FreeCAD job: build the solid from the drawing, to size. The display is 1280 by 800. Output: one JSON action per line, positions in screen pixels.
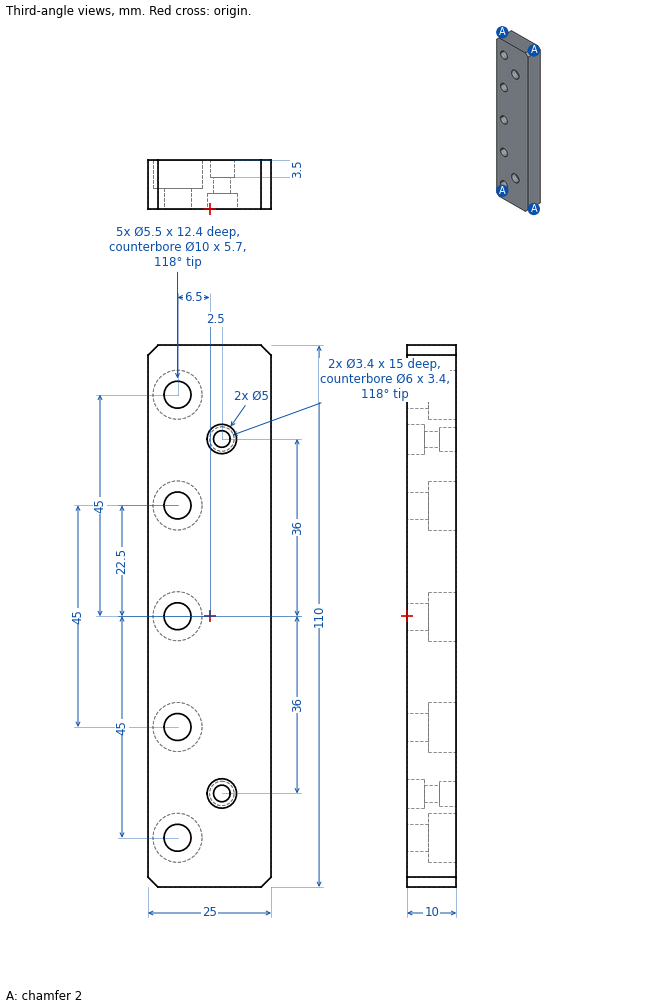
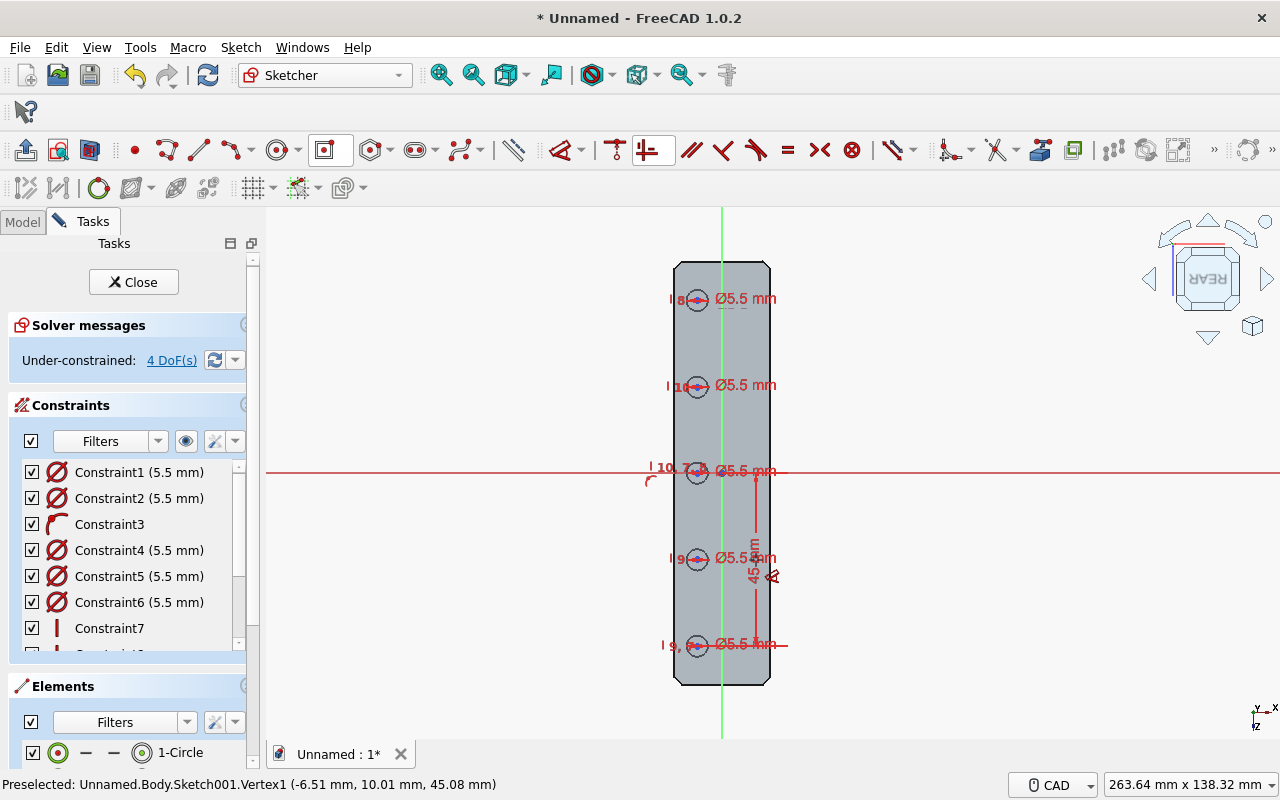
{"action": "left_click", "coordinate": [697, 301]}
{"action": "left_click", "coordinate": [756, 387]}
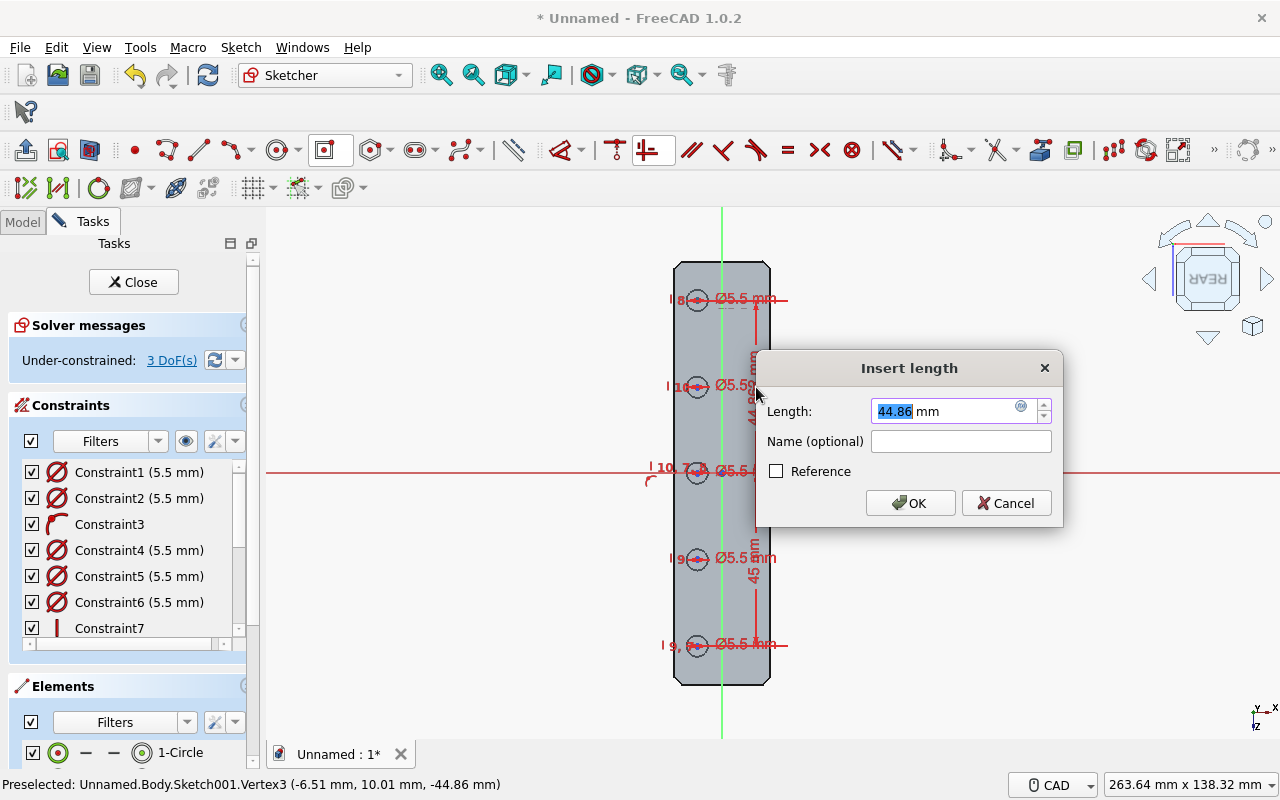
{"action": "type", "text": "45"}
{"action": "key", "text": "Return"}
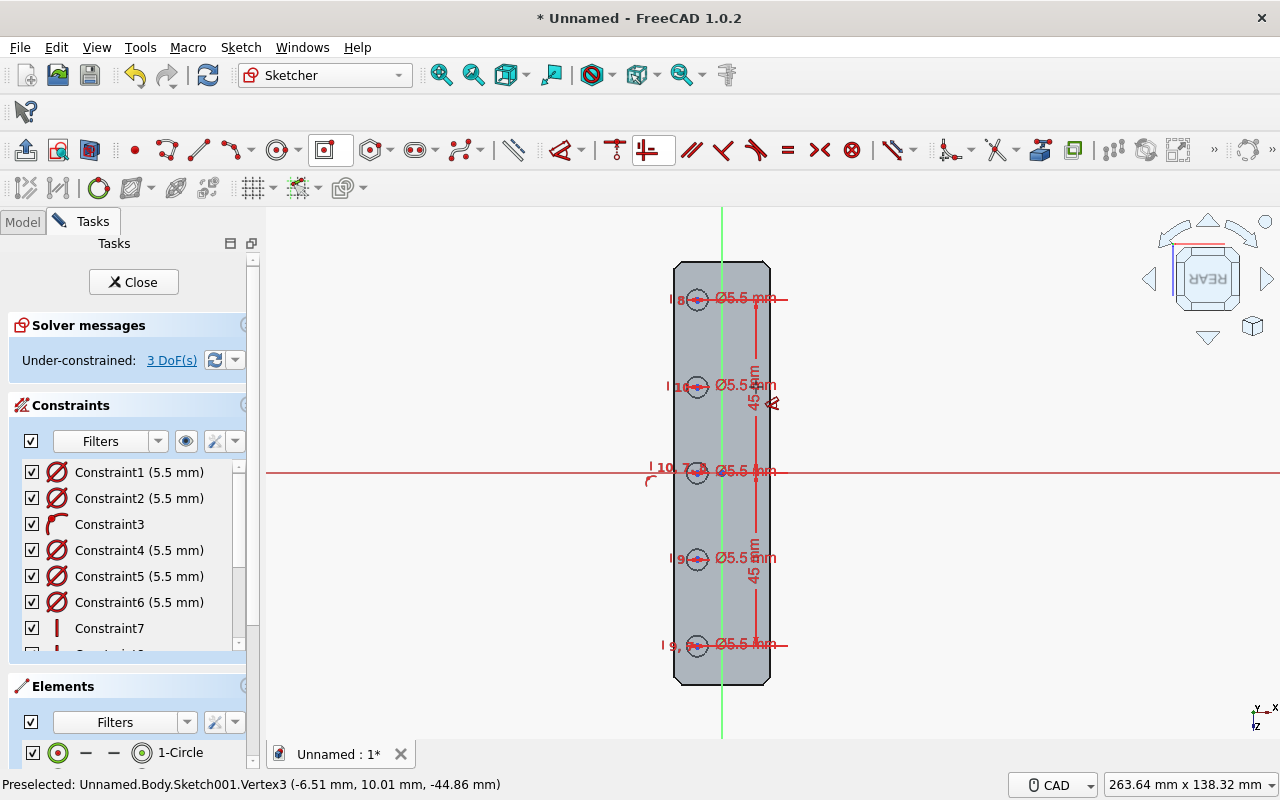
{"action": "scroll", "coordinate": [697, 646], "scroll_direction": "up", "scroll_amount": 3}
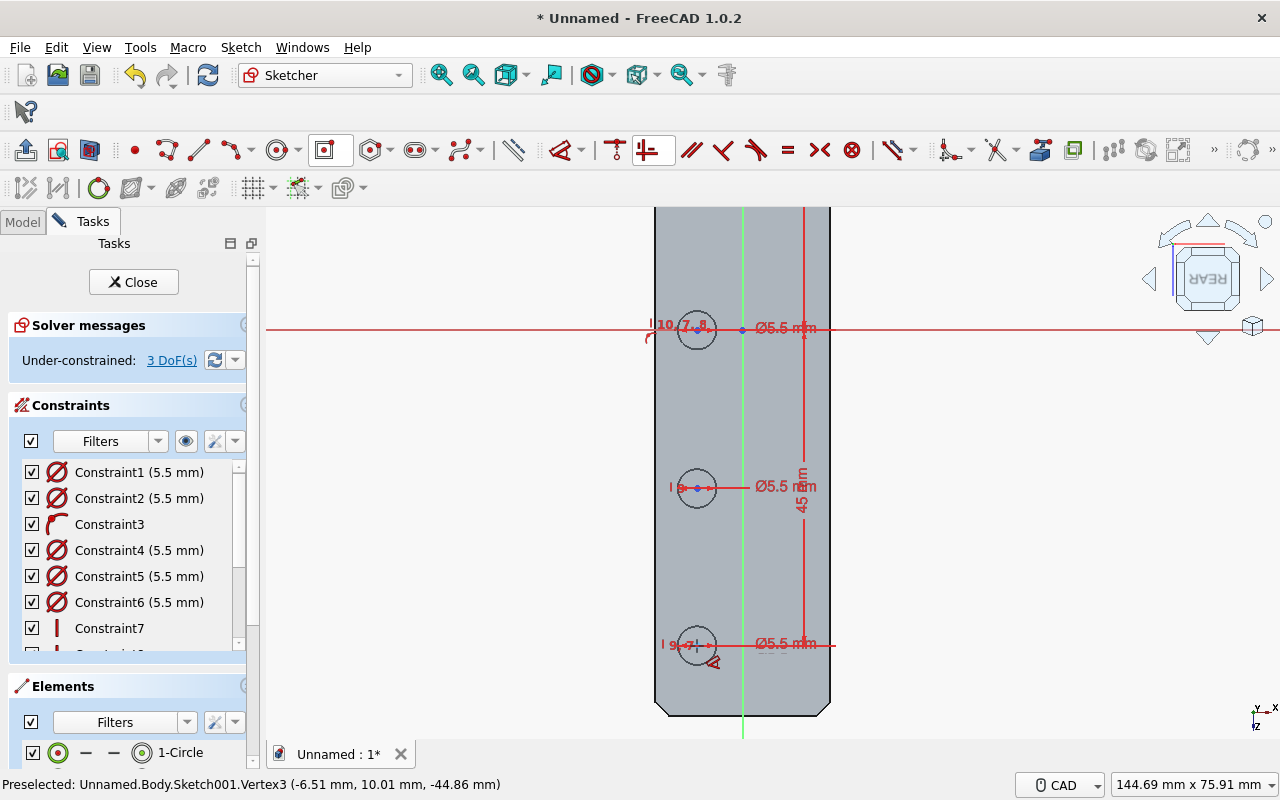
{"action": "left_click", "coordinate": [697, 646]}
{"action": "left_click", "coordinate": [720, 680]}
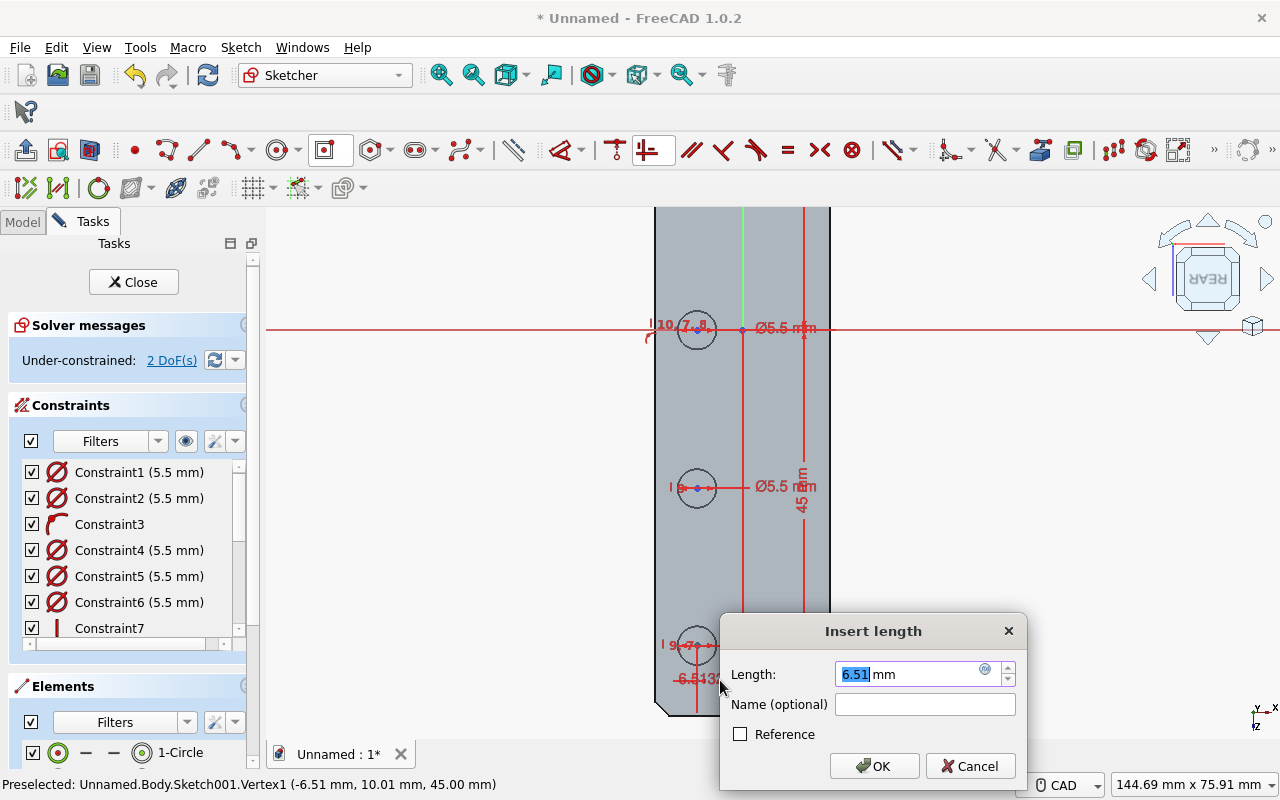
{"action": "type", "text": "6.5"}
{"action": "key", "text": "Return"}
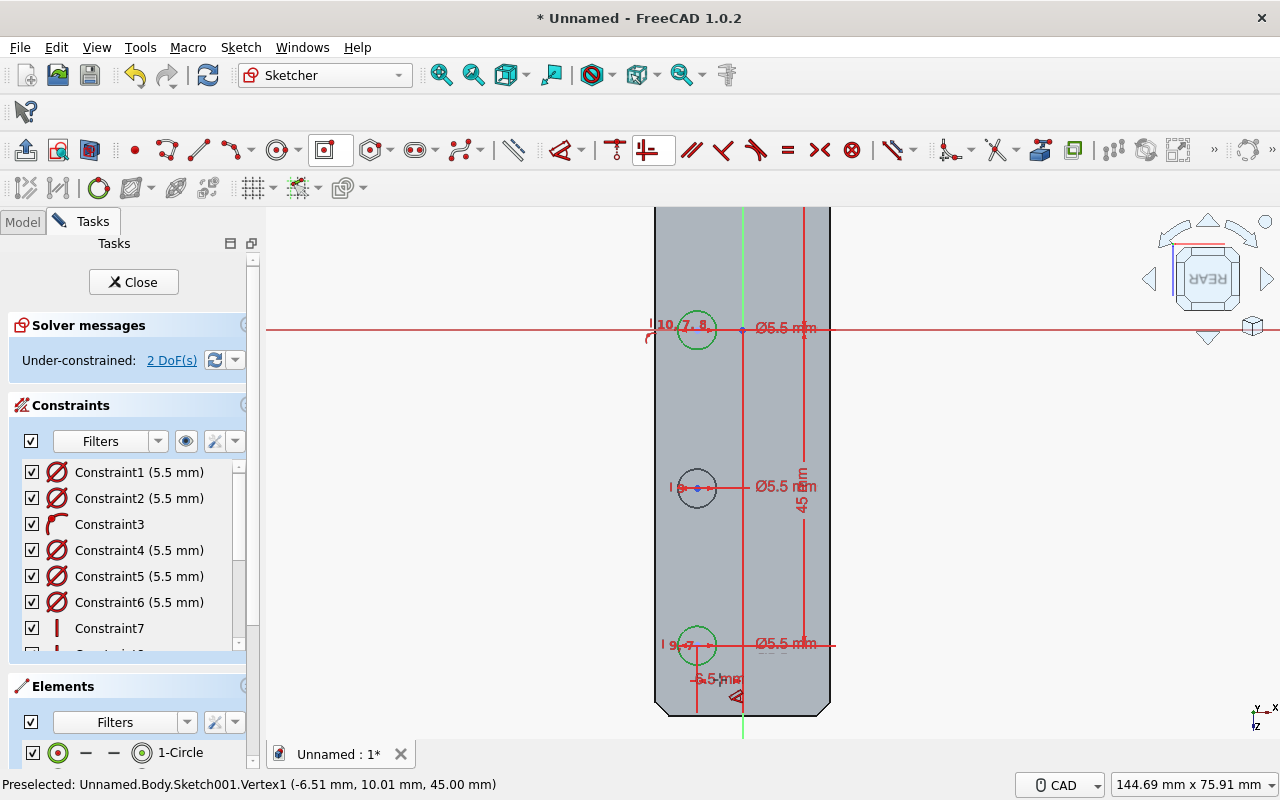
{"action": "left_click", "coordinate": [697, 488]}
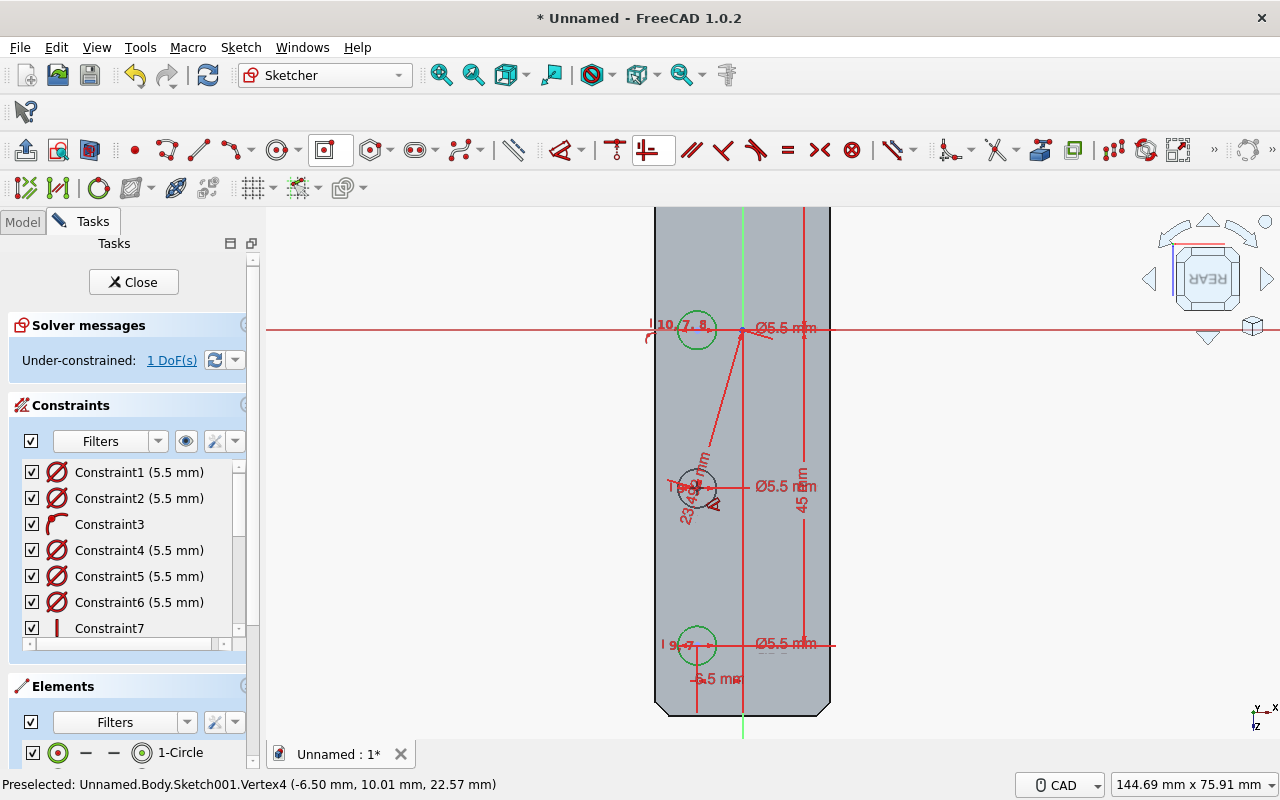
{"action": "scroll", "coordinate": [697, 647], "scroll_direction": "down", "scroll_amount": 3}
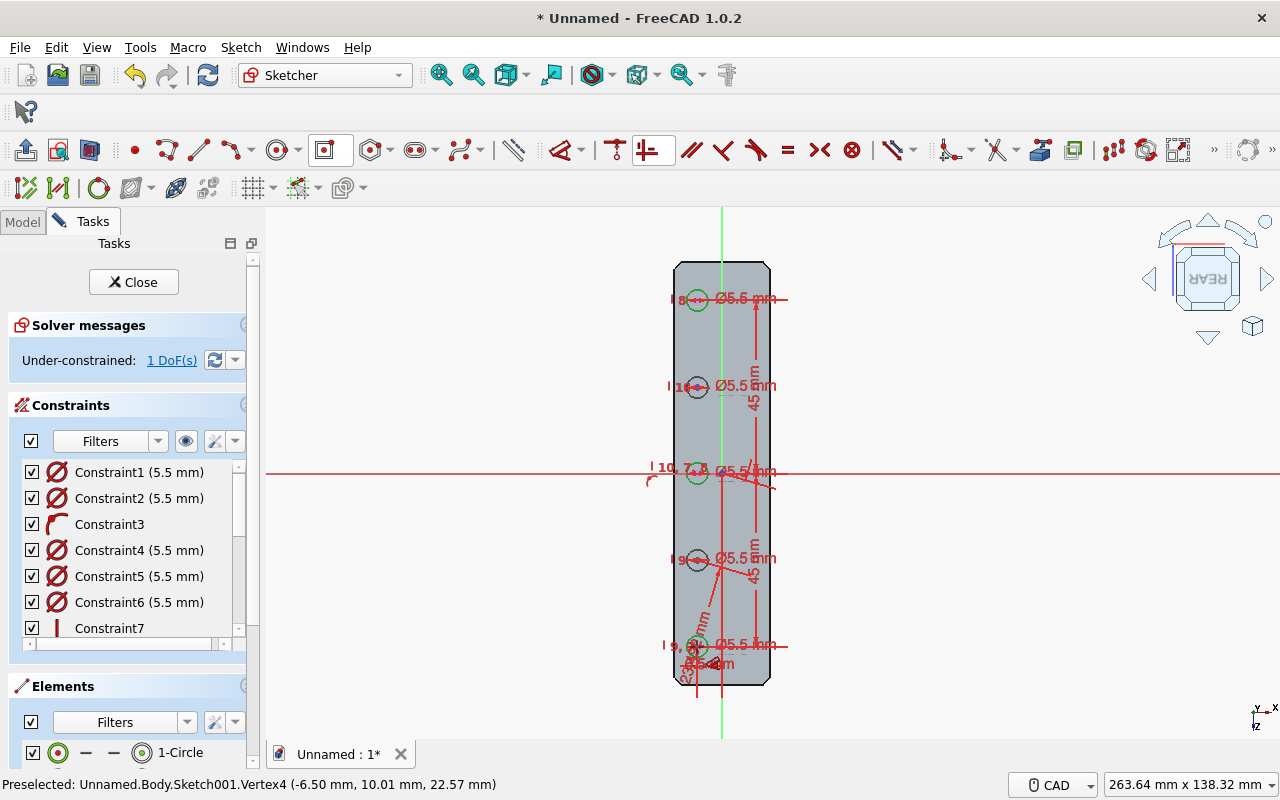
{"action": "left_click", "coordinate": [697, 388]}
{"action": "left_click", "coordinate": [663, 434]}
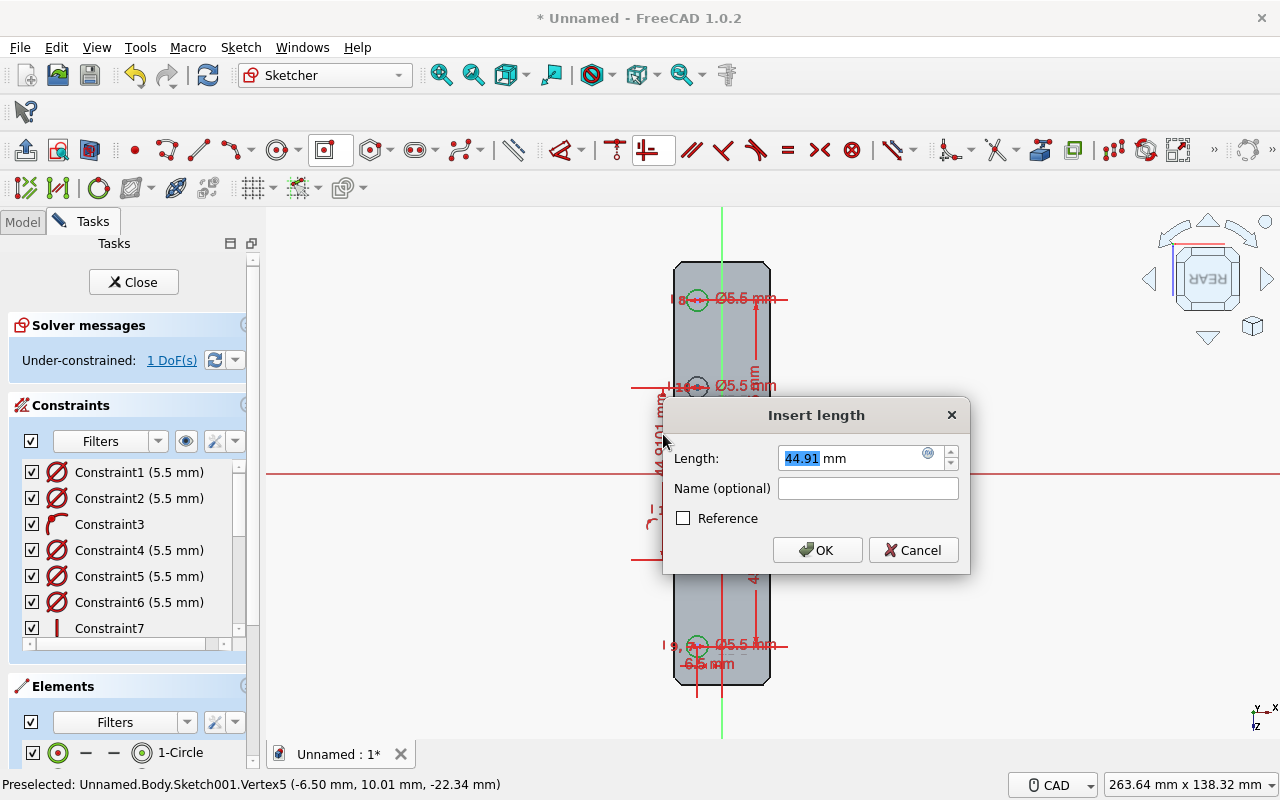
{"action": "type", "text": "45"}
{"action": "key", "text": "Return"}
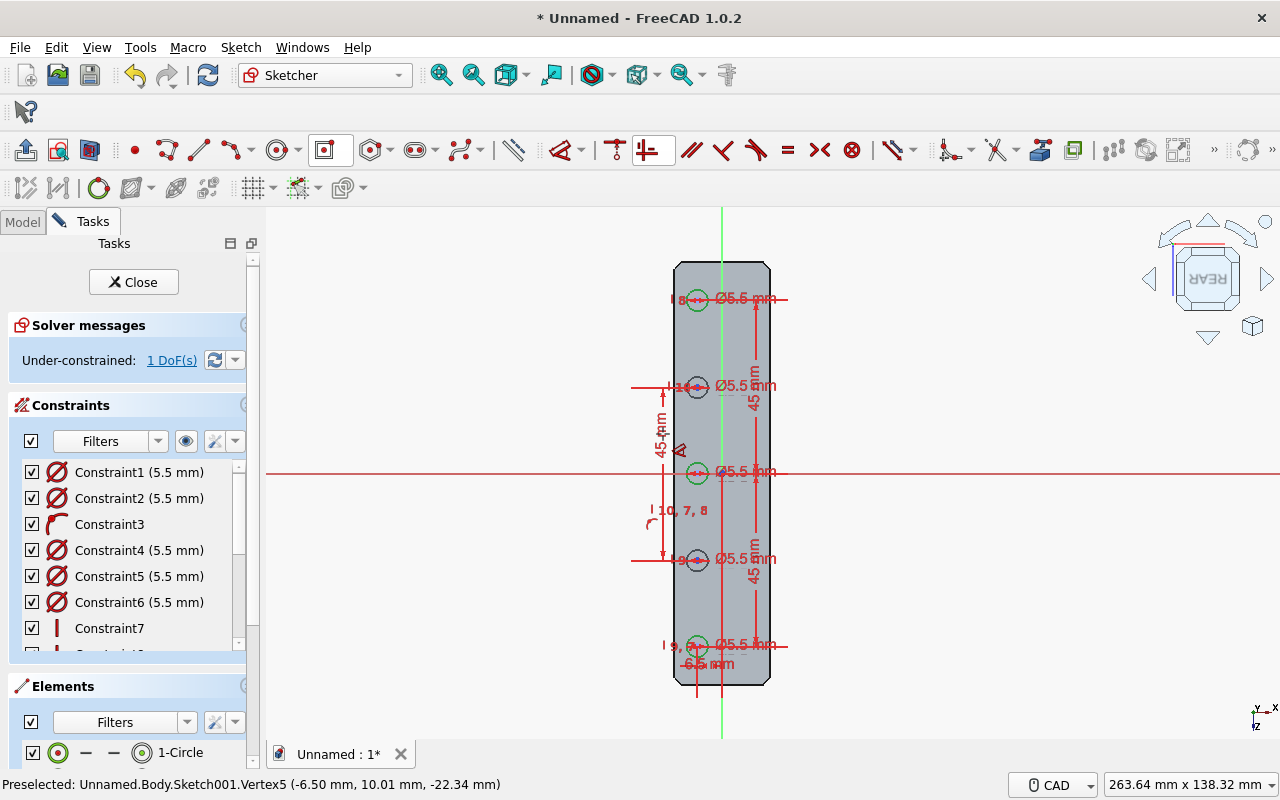
{"action": "left_click", "coordinate": [697, 561]}
{"action": "left_click", "coordinate": [756, 517]}